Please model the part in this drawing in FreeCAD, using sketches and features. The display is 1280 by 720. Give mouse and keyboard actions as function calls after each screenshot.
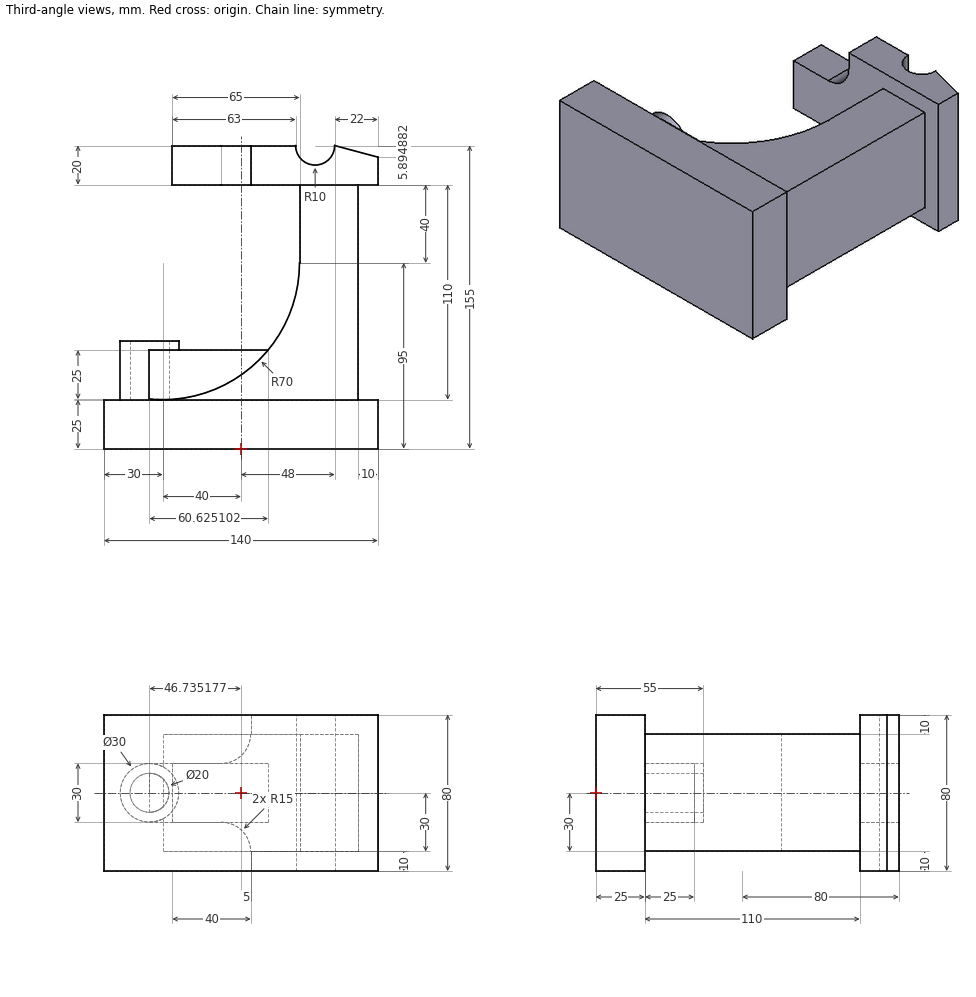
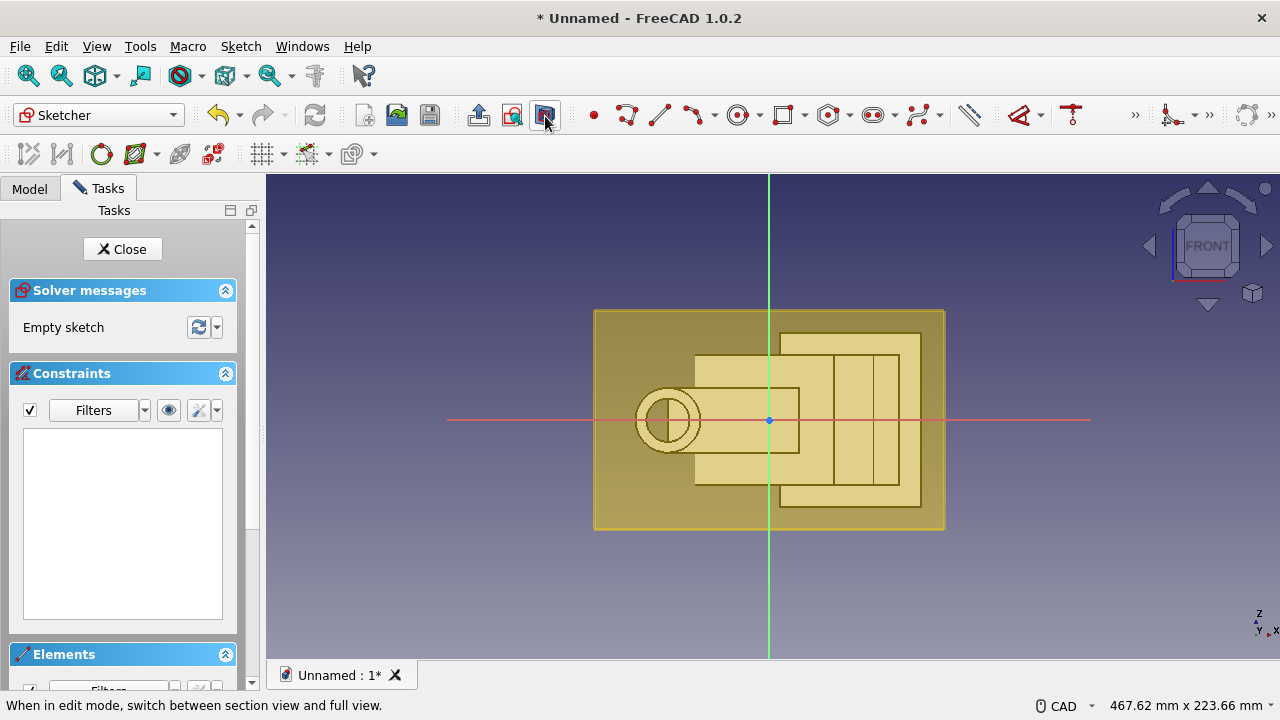
scroll(662, 421, up, 10)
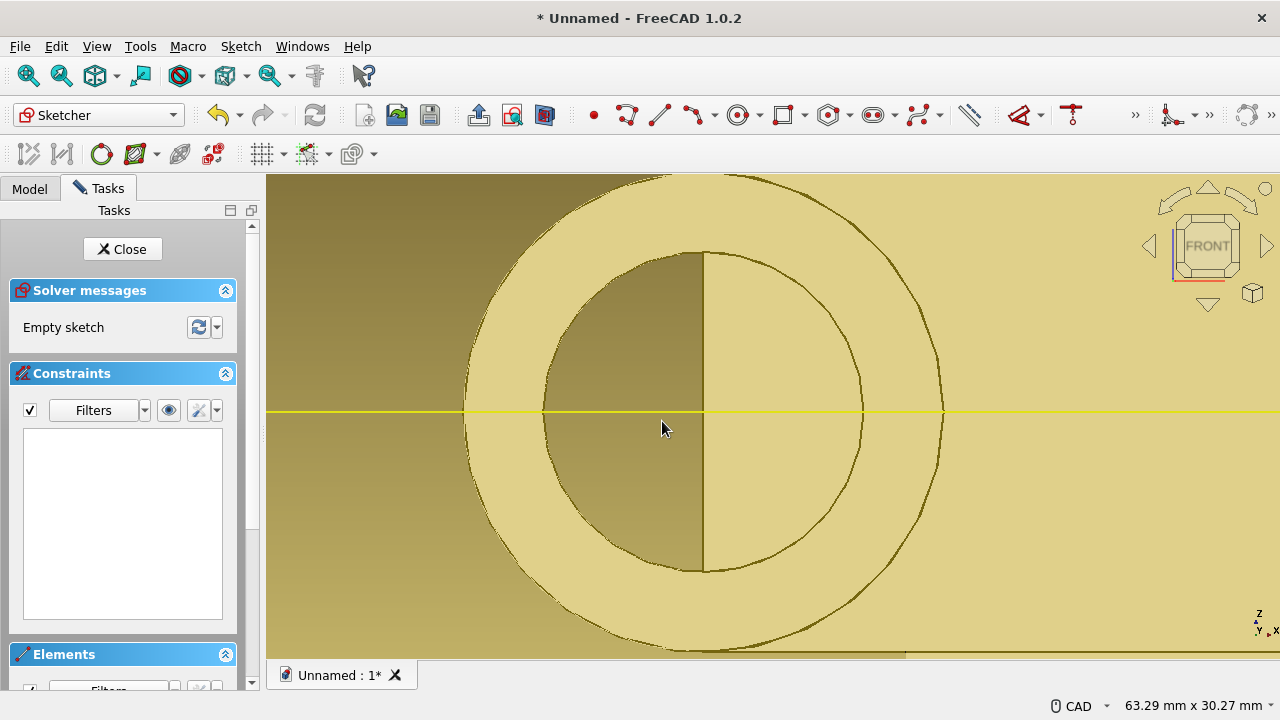
click(738, 116)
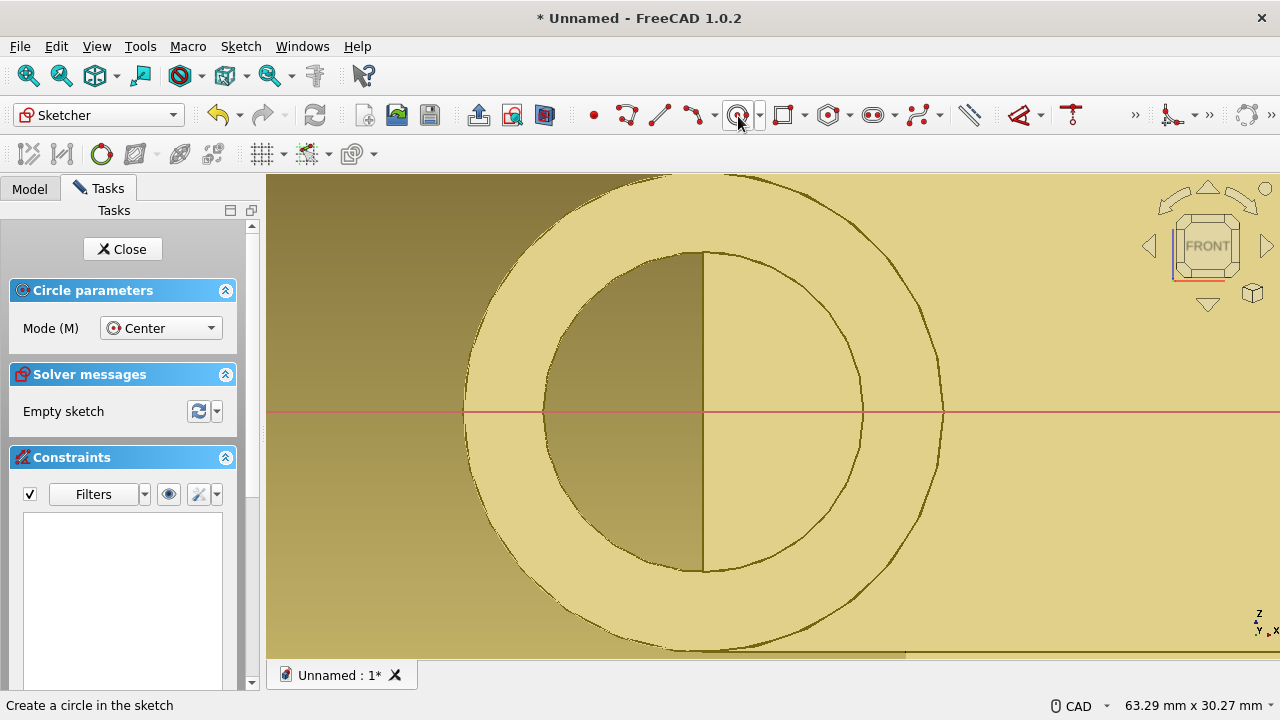
click(703, 412)
move(817, 299)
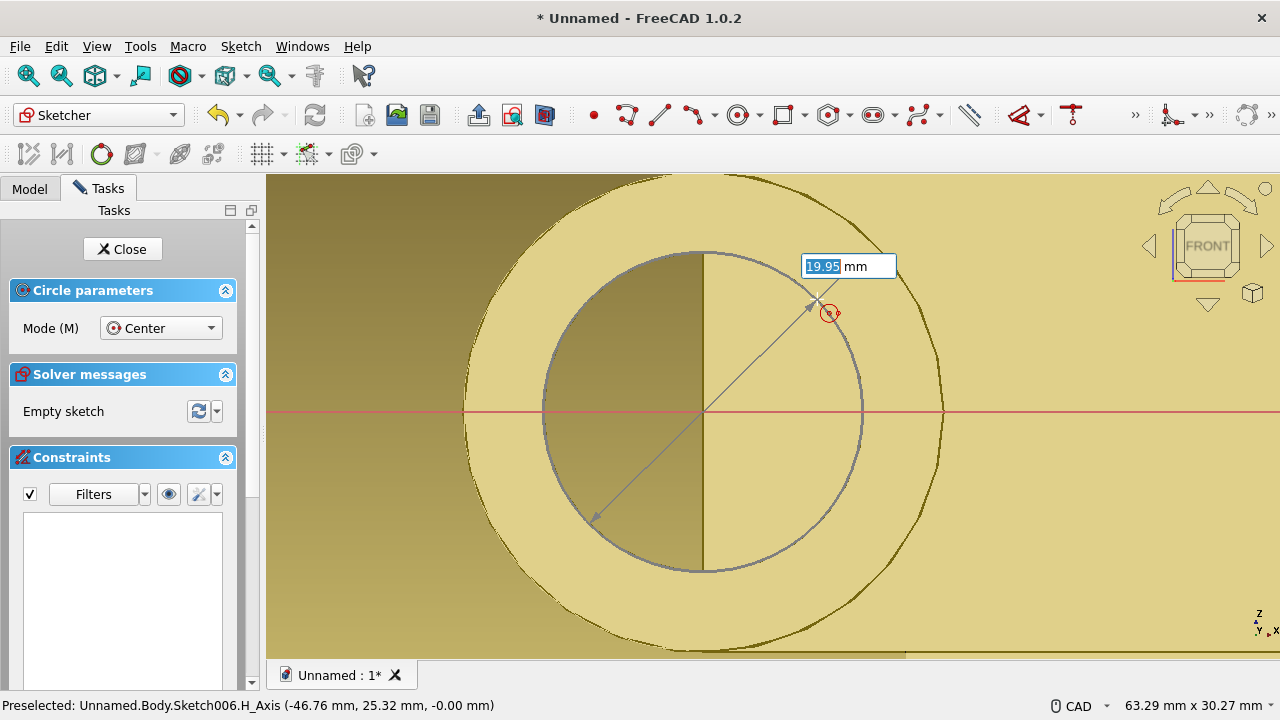
text(20)
key(Return)
key(Escape)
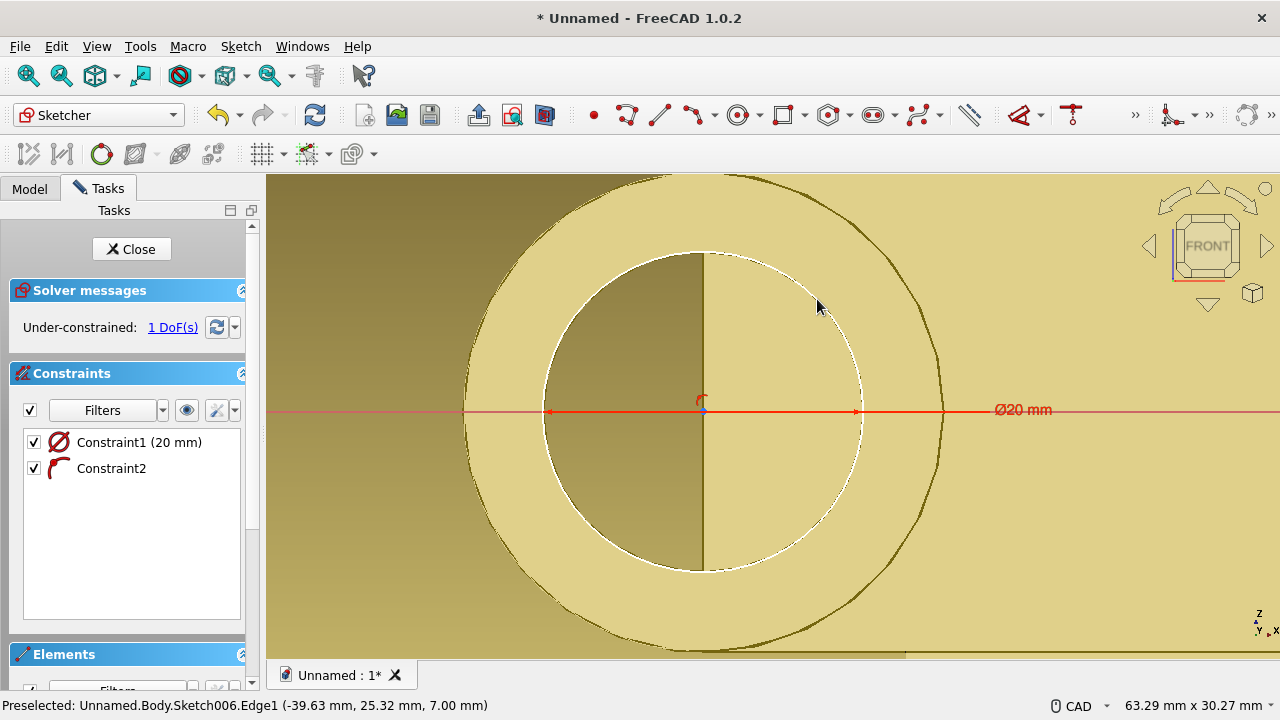
click(1018, 116)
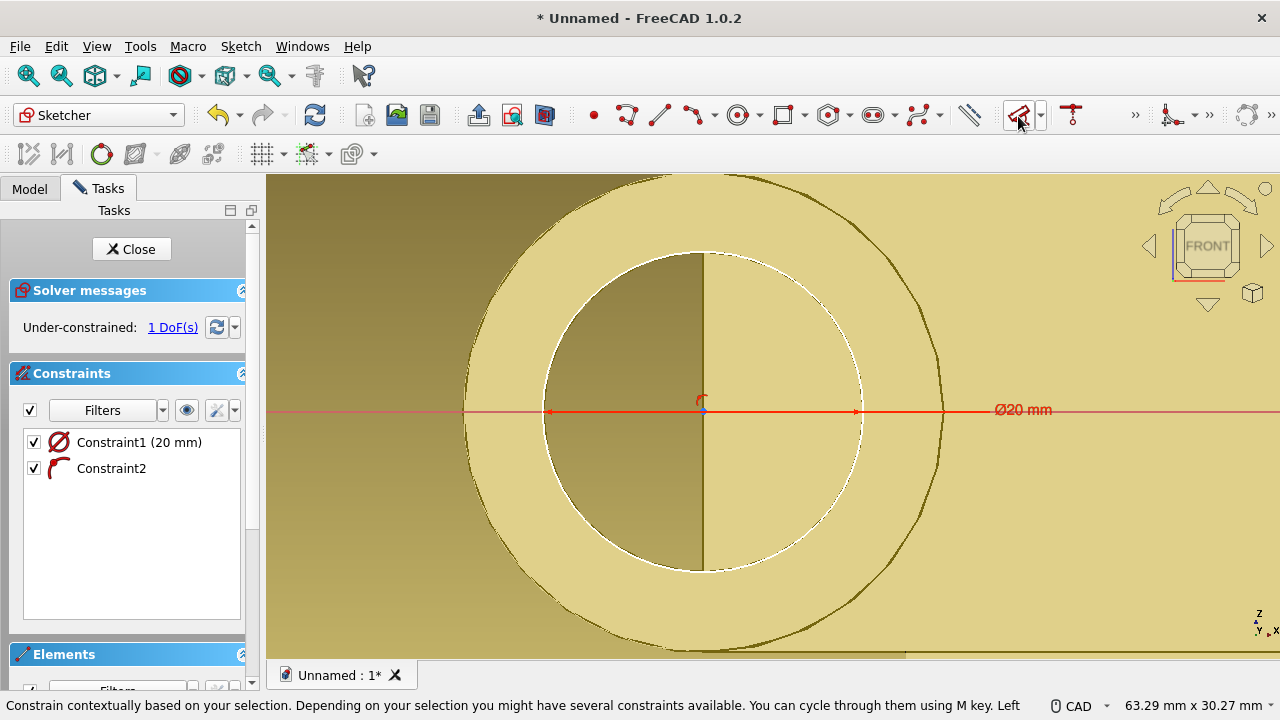
click(703, 412)
click(909, 446)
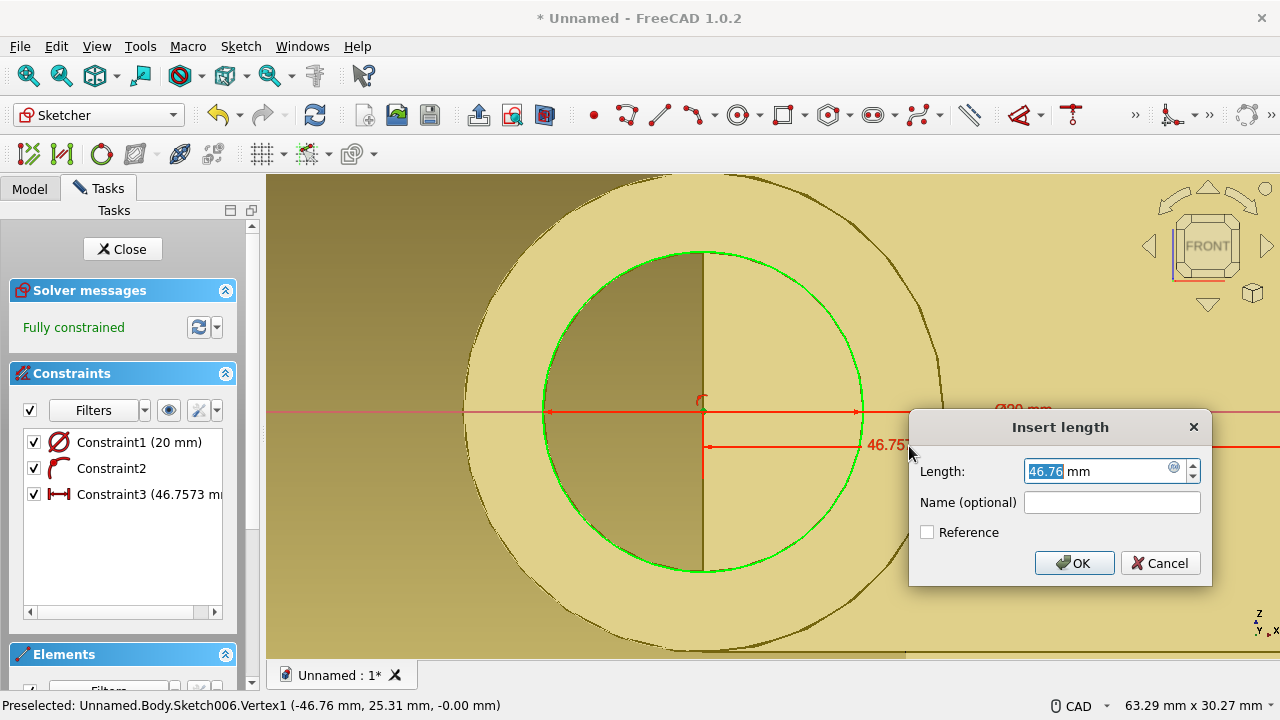
text(46.735177)
key(Return)
key(Escape)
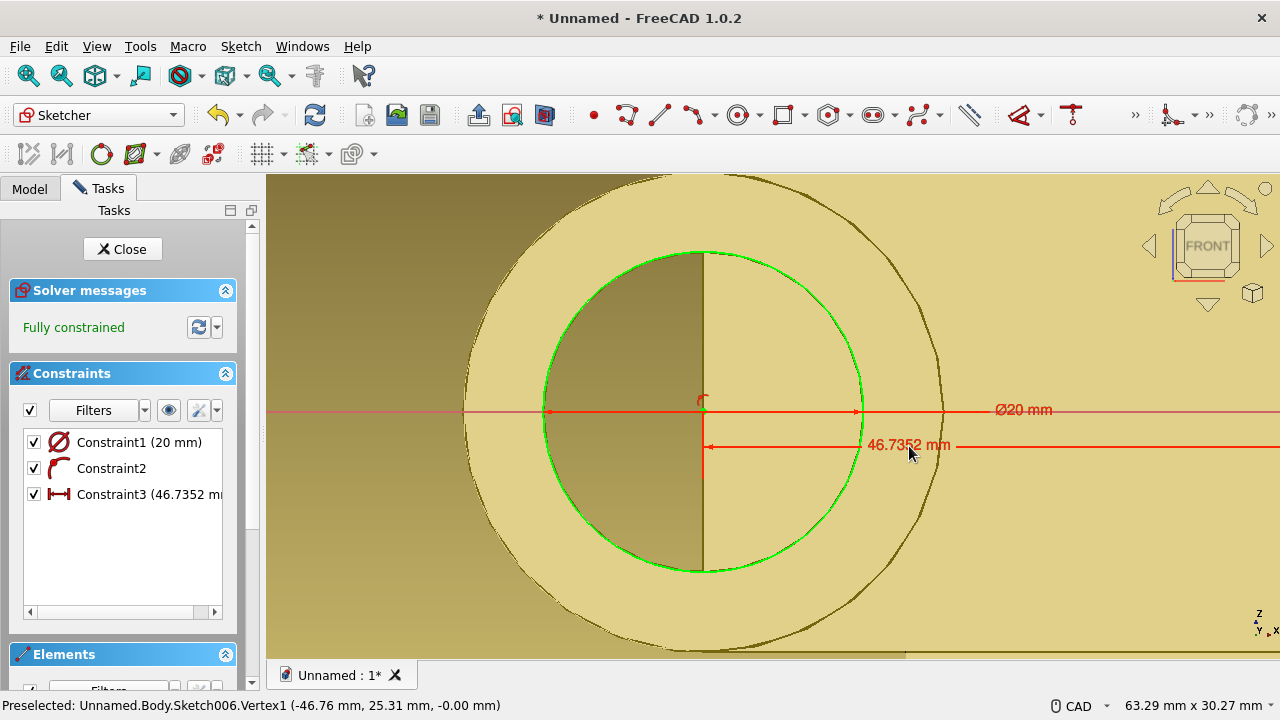
click(123, 249)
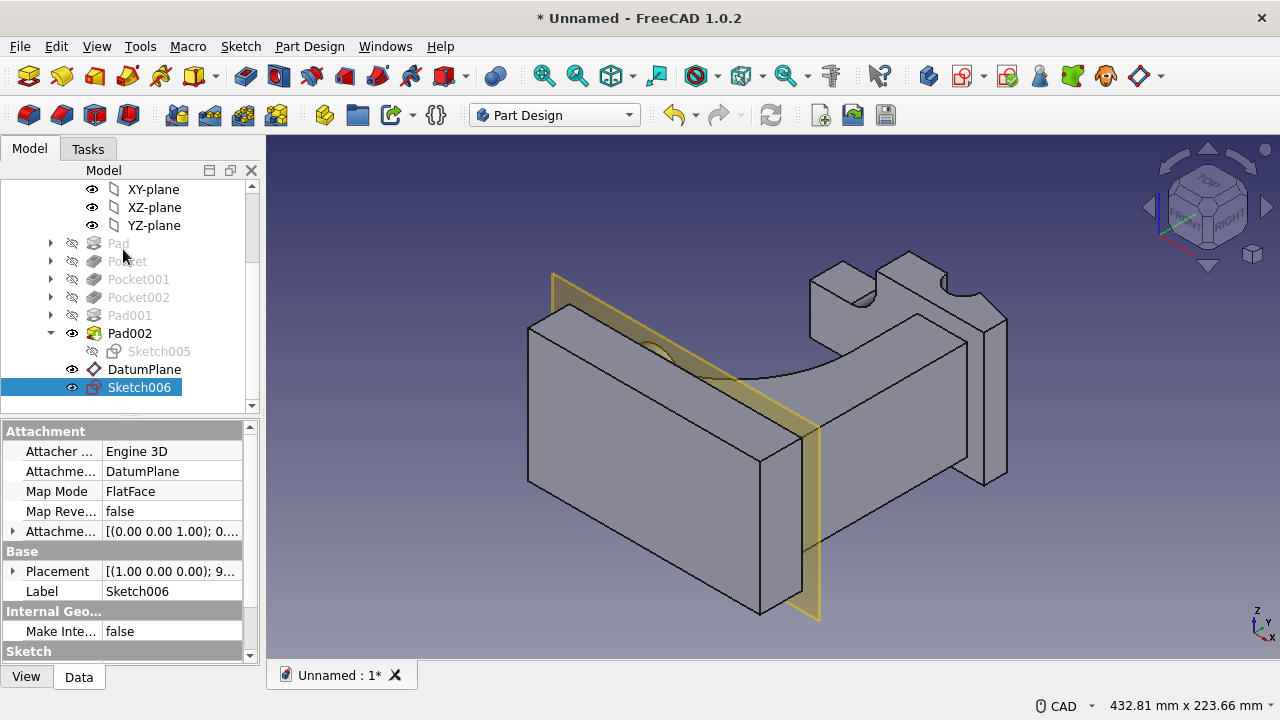
click(246, 76)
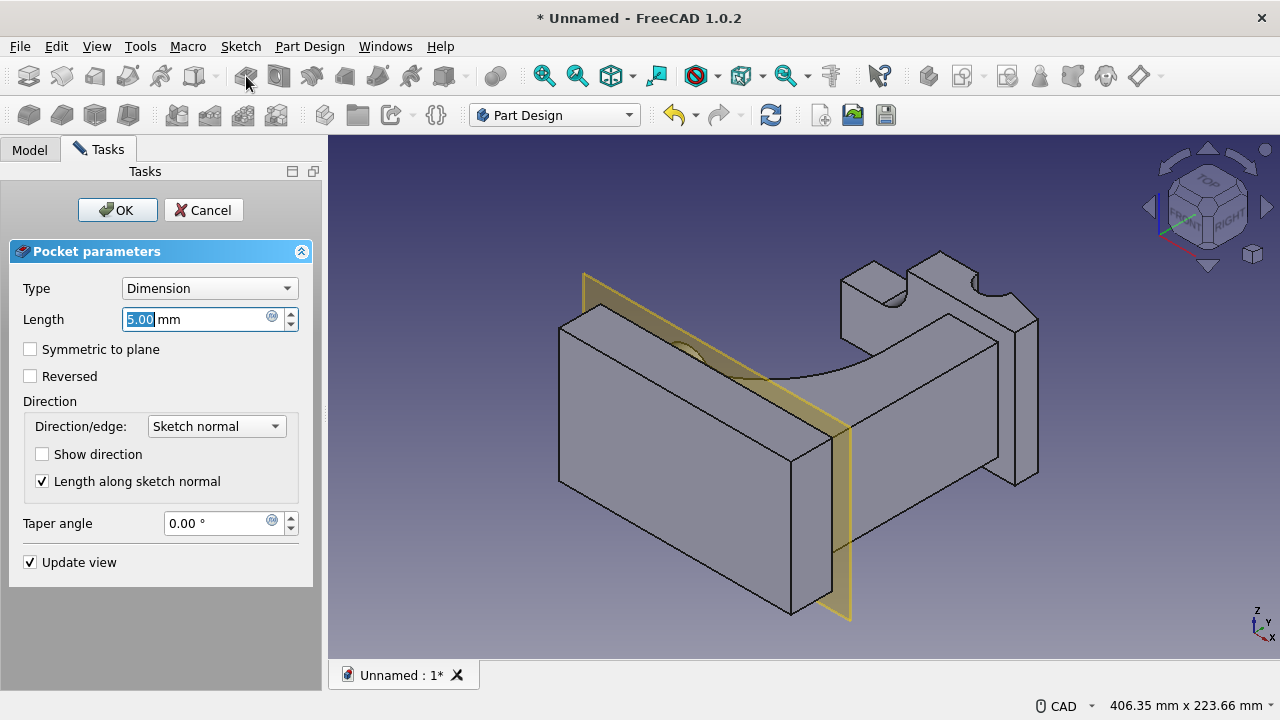
text(25)
key(Tab)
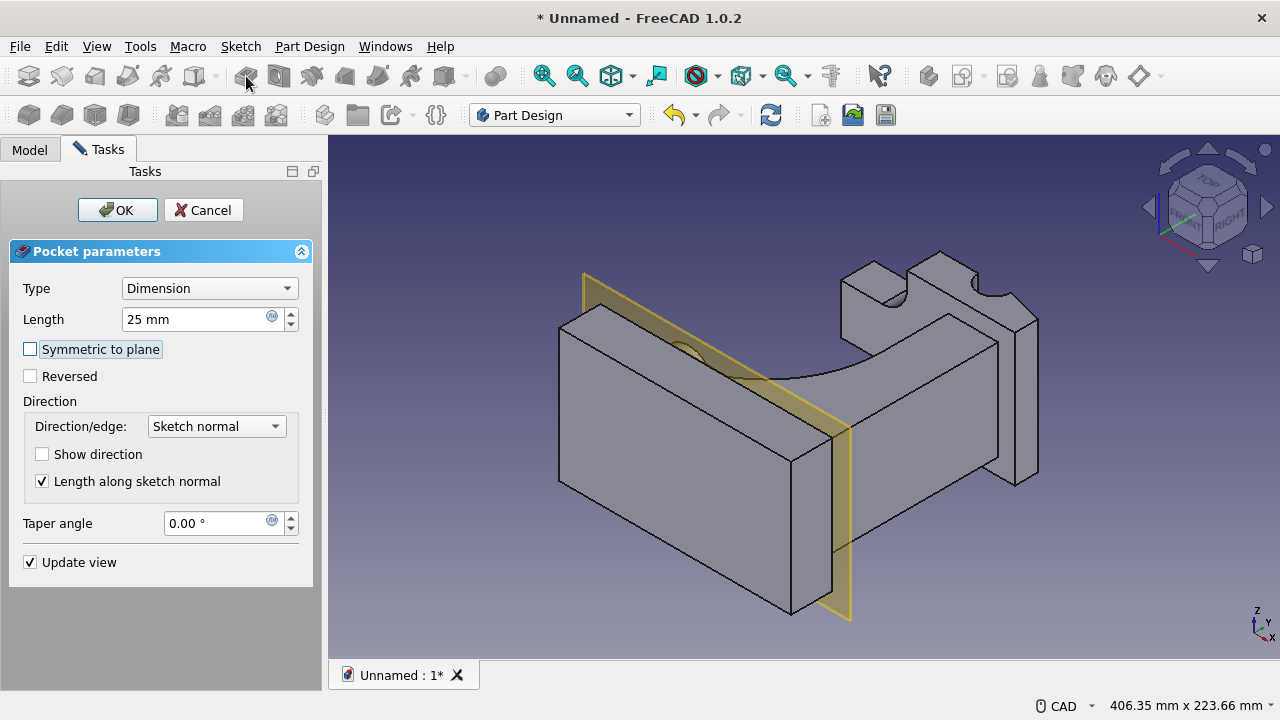
click(118, 210)